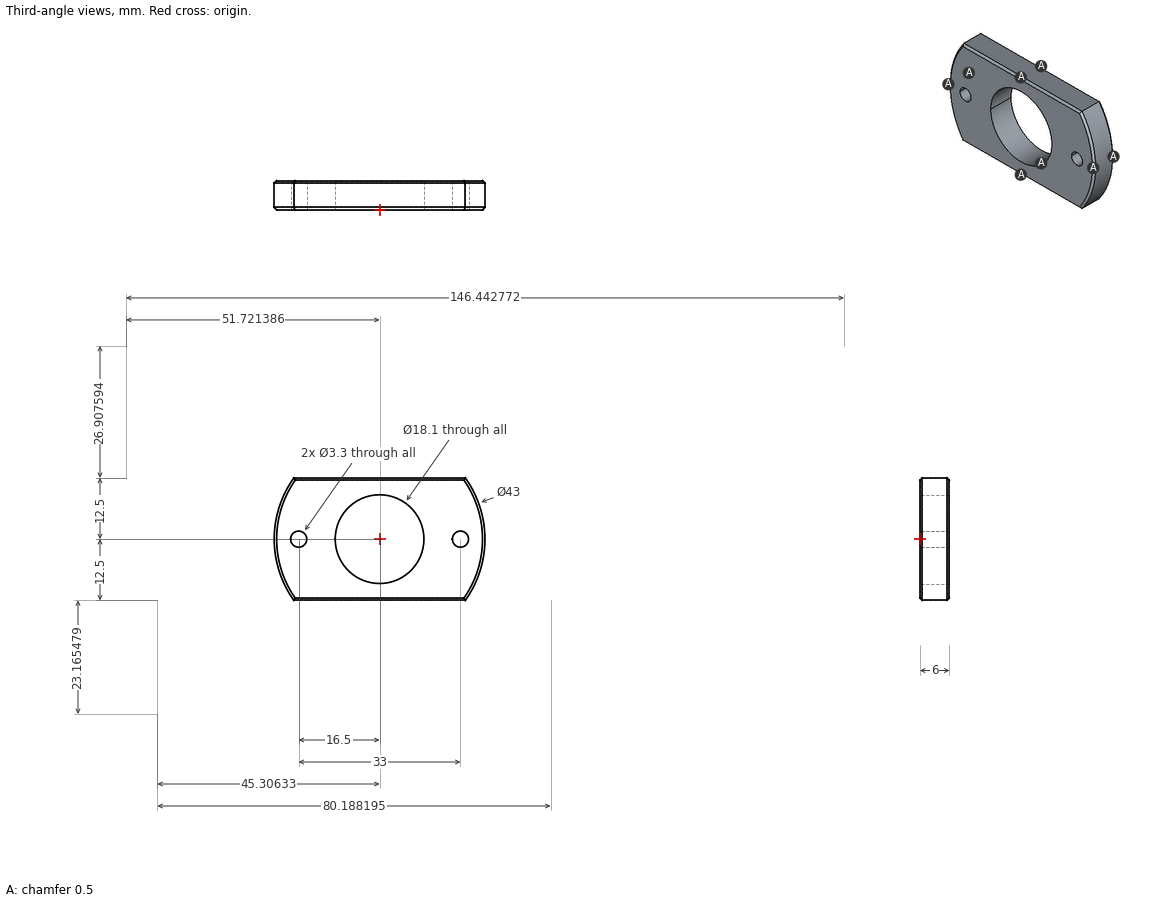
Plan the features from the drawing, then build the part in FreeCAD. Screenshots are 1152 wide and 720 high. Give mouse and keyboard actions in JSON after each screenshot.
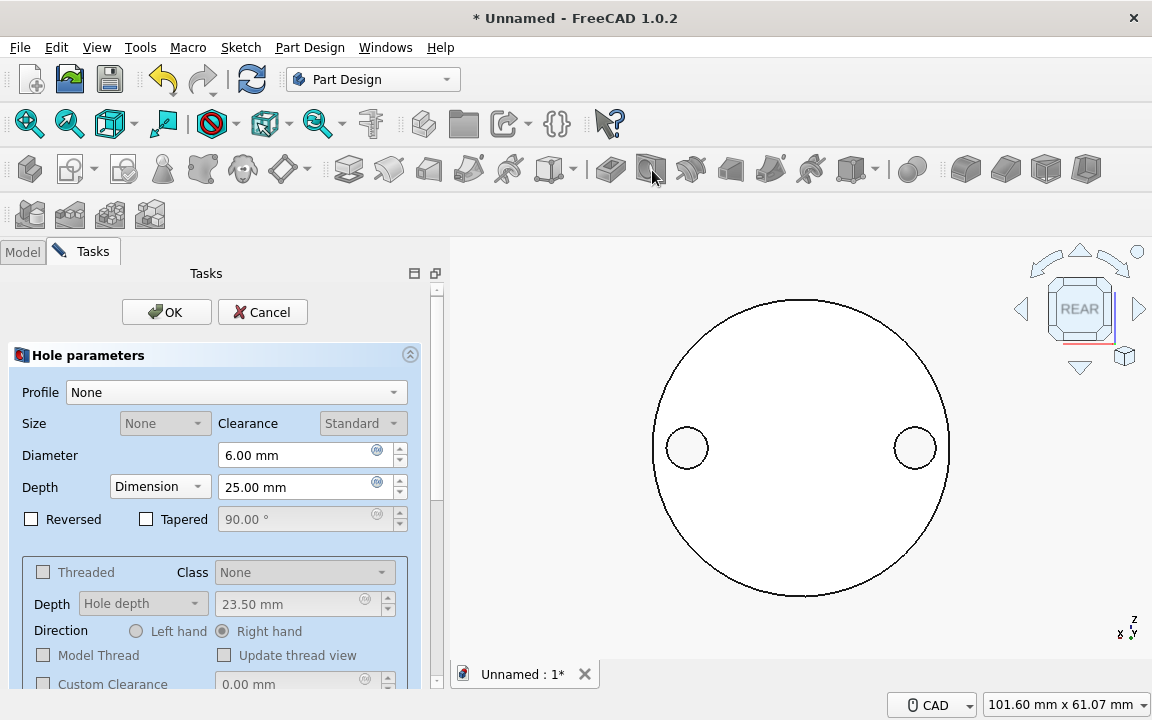
{"action": "triple_click", "coordinate": [305, 455]}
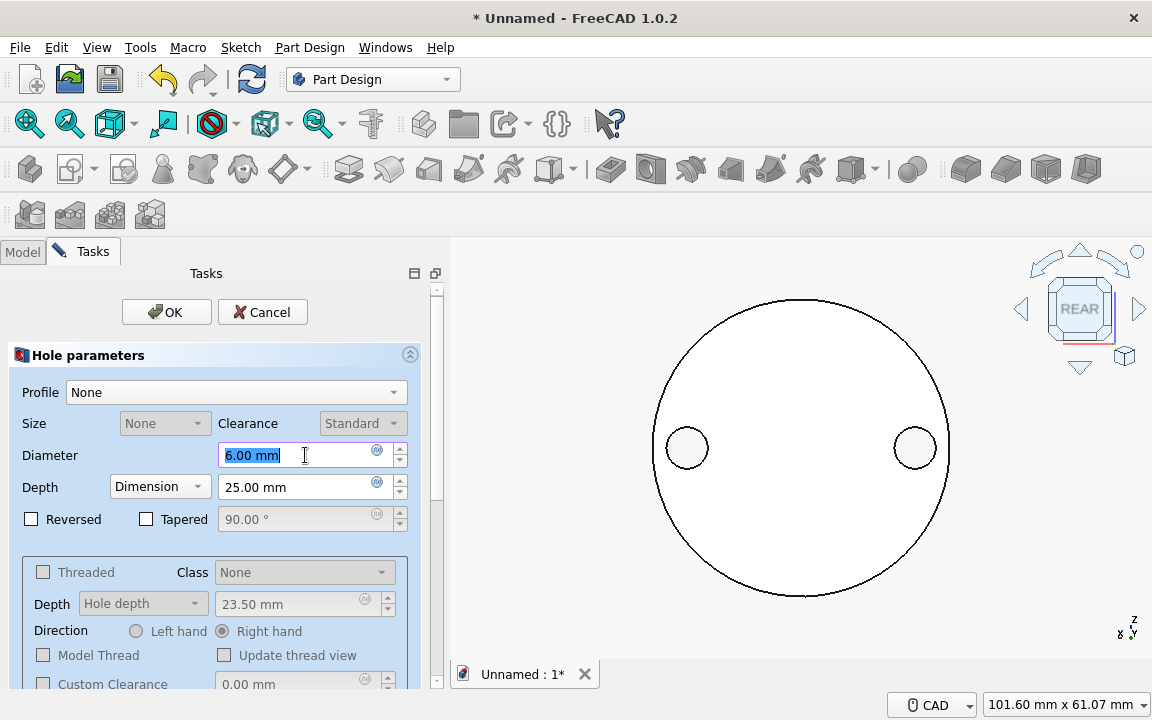
{"action": "type", "text": "3.3"}
{"action": "key", "text": "Tab"}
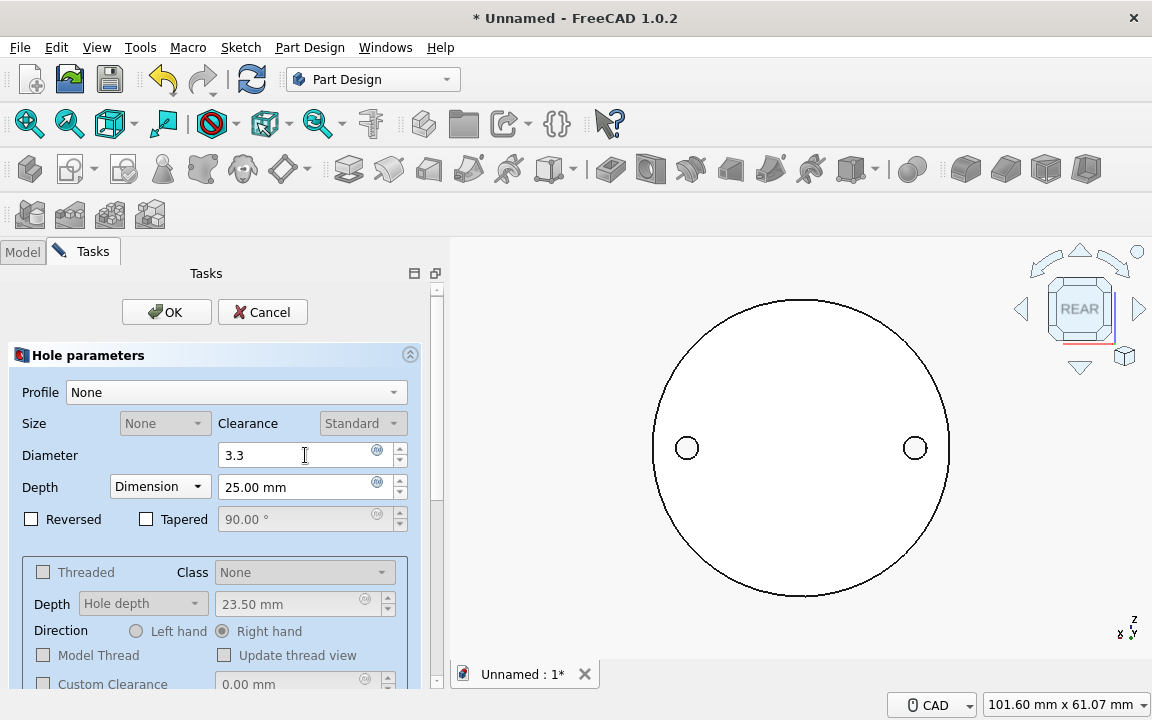
{"action": "left_click", "coordinate": [161, 486]}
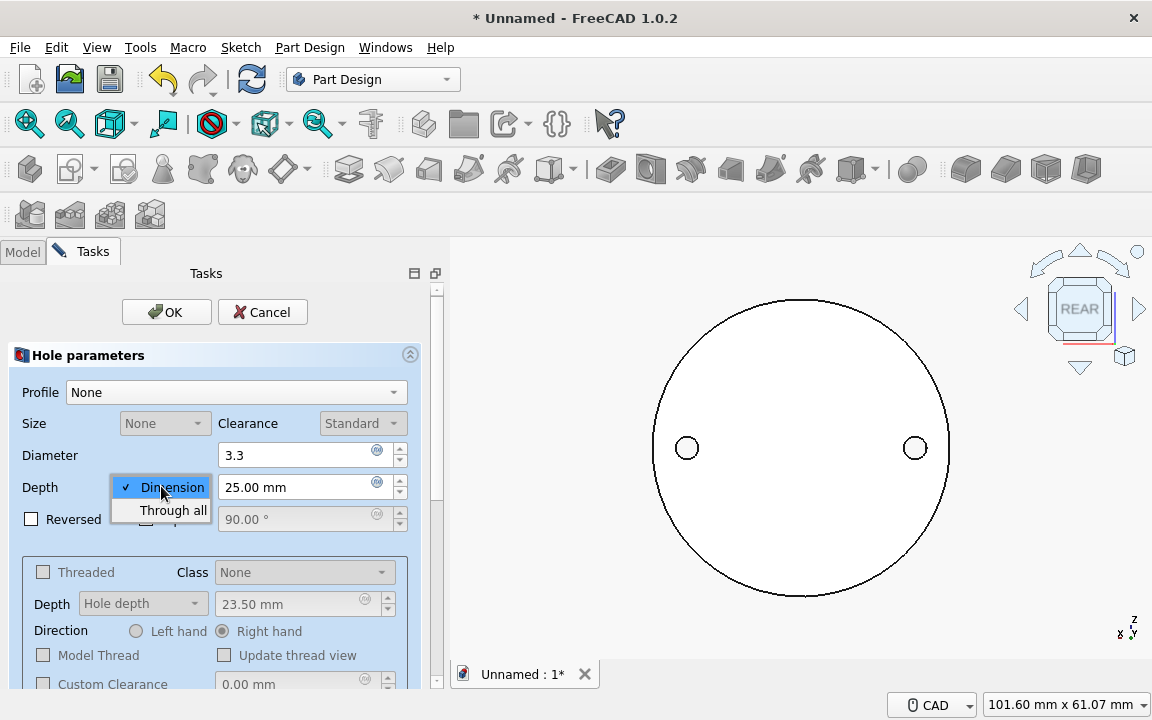
{"action": "left_click", "coordinate": [160, 510]}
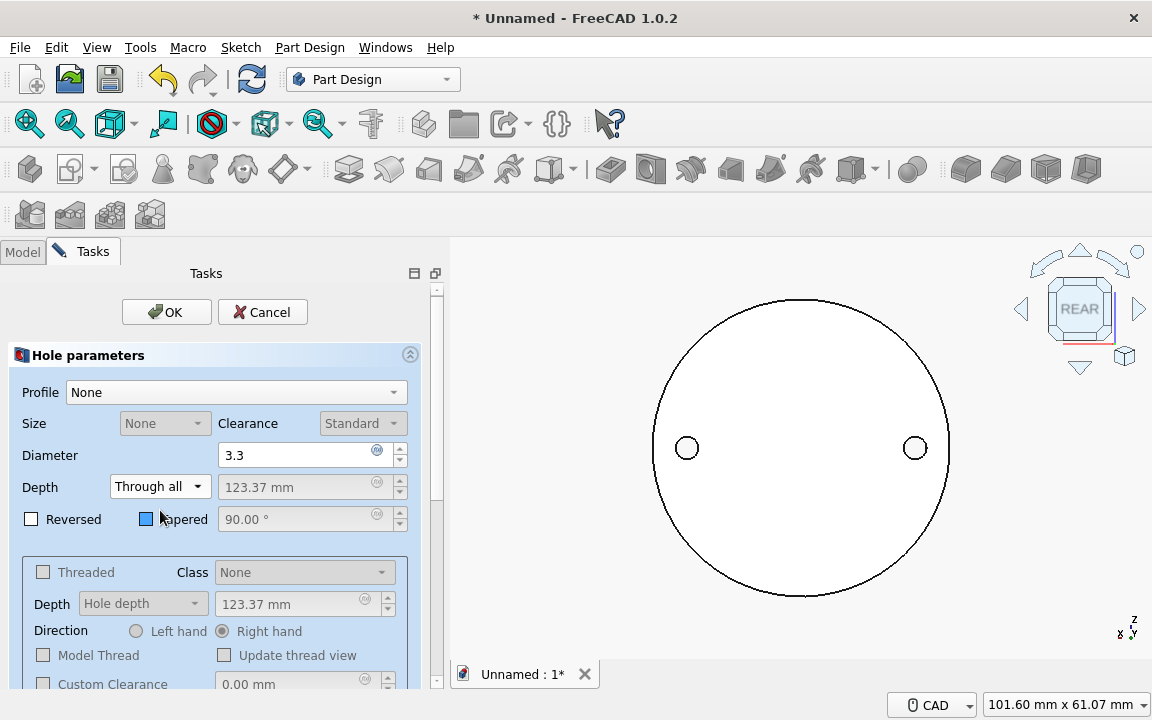
{"action": "left_click", "coordinate": [167, 312]}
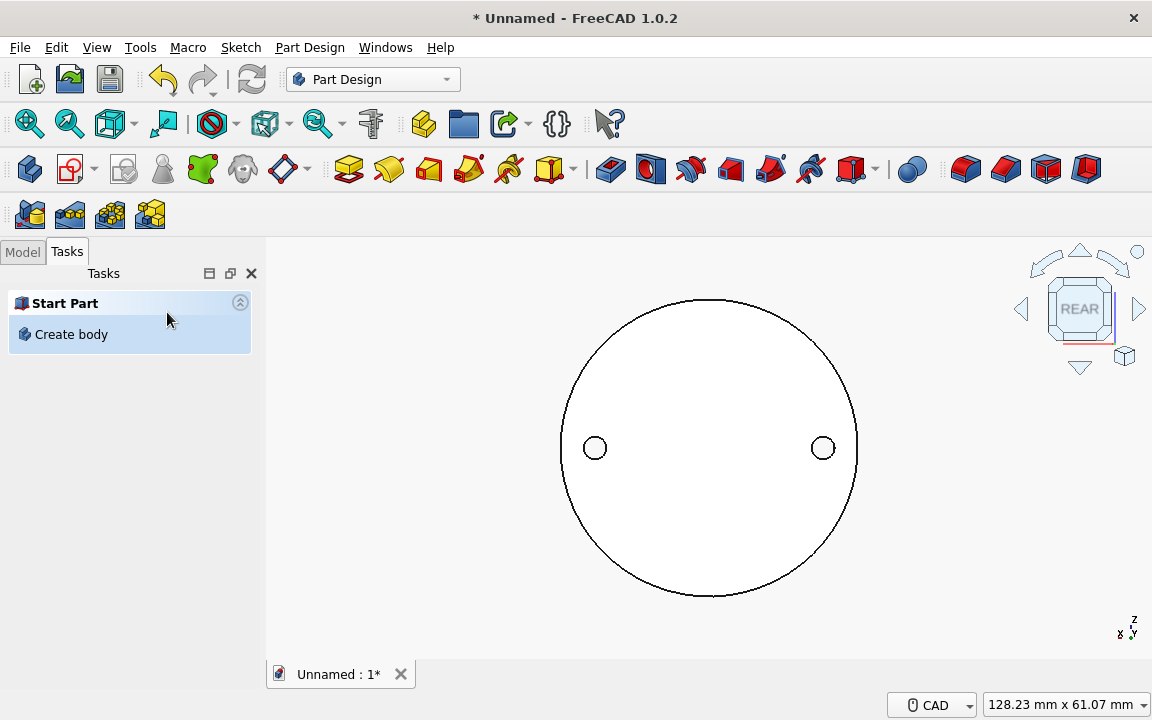
{"action": "left_click", "coordinate": [709, 405]}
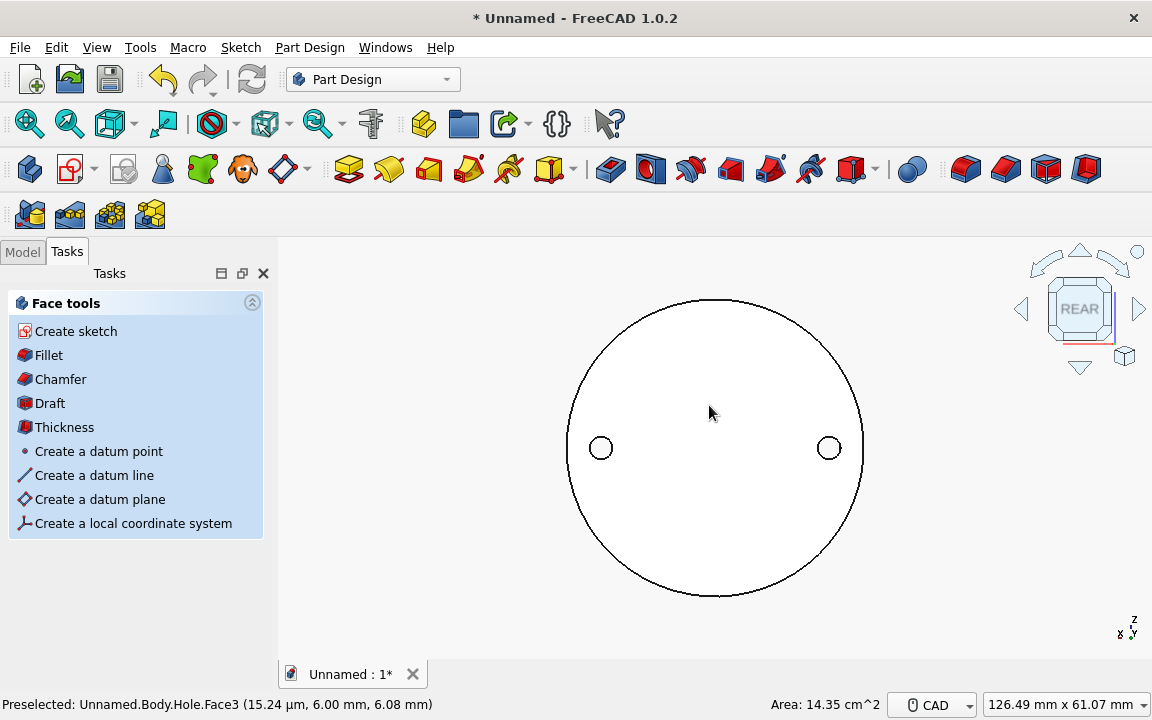
{"action": "left_click", "coordinate": [70, 170]}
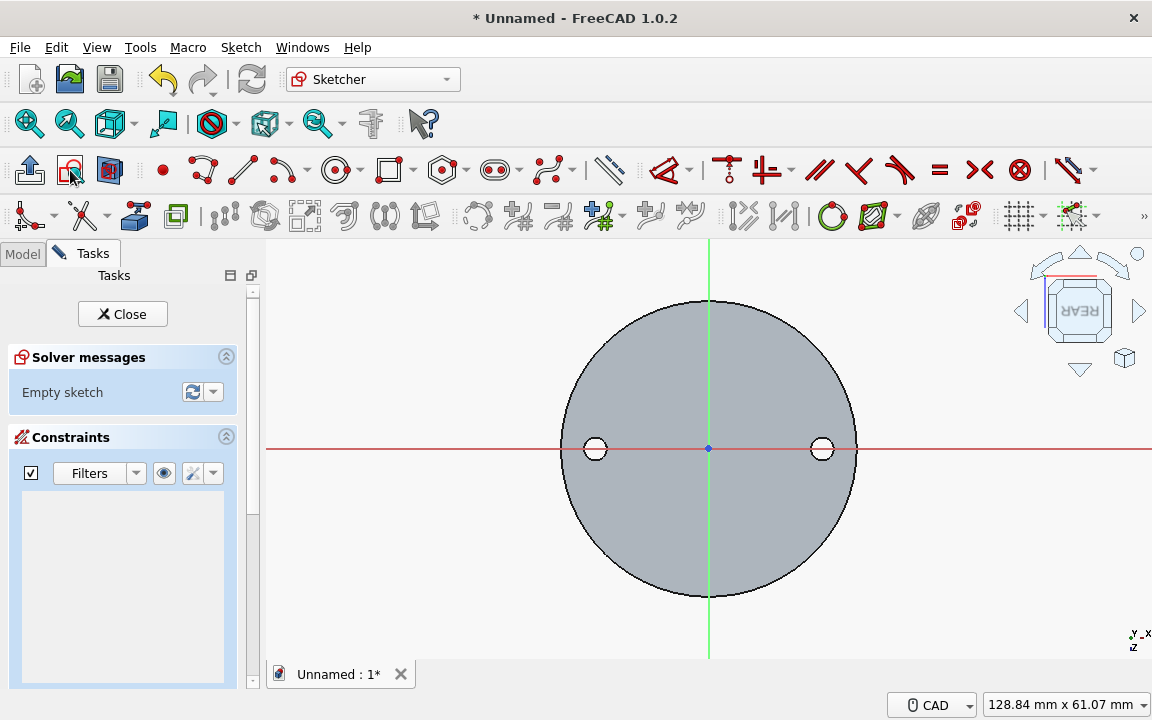
{"action": "scroll", "coordinate": [464, 439], "scroll_direction": "down", "scroll_amount": 4}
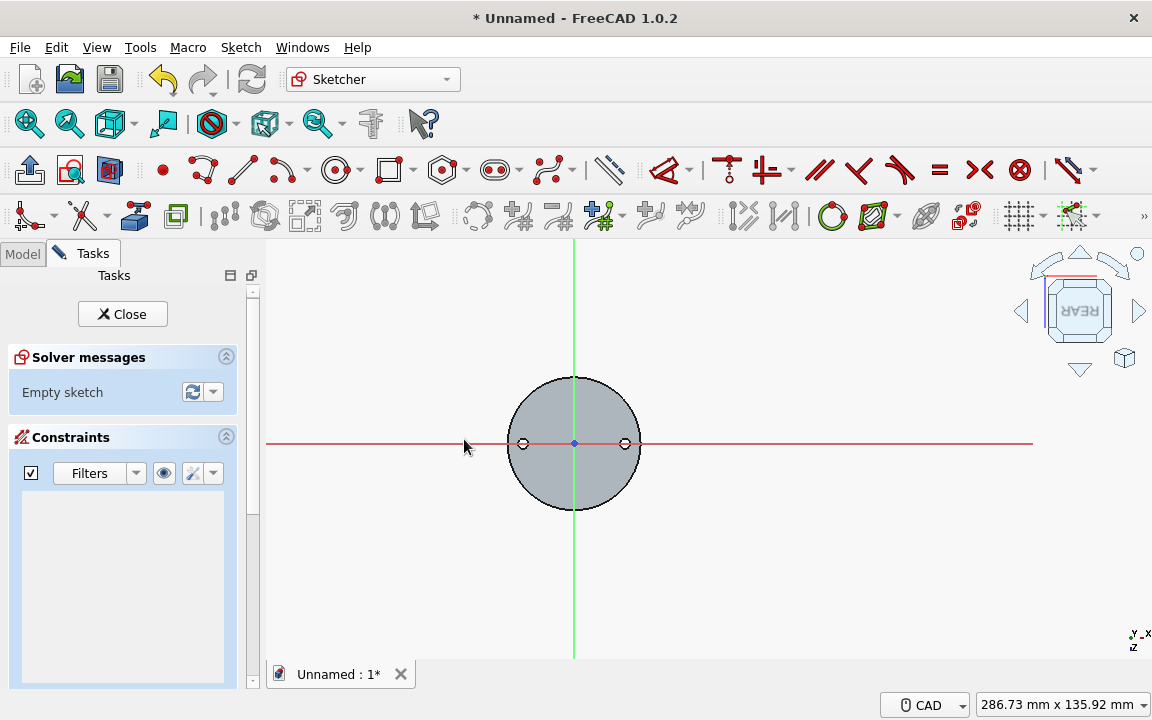
{"action": "left_click", "coordinate": [390, 170]}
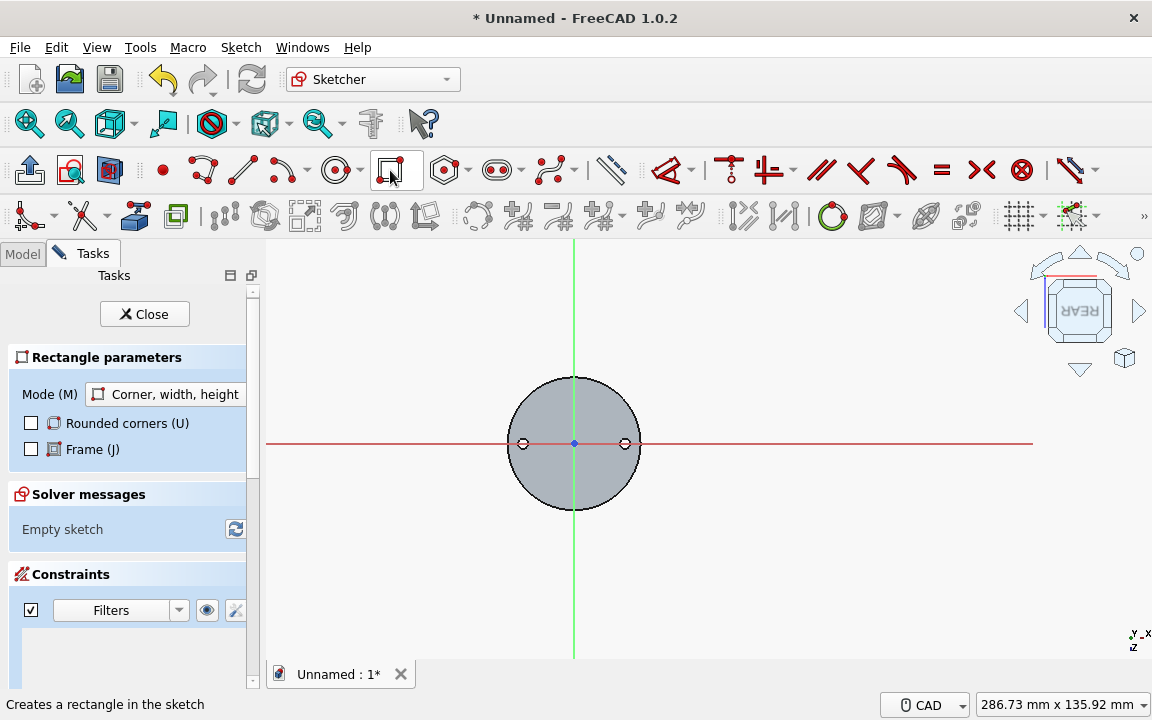
{"action": "left_click", "coordinate": [434, 334]}
{"action": "left_click", "coordinate": [682, 405]}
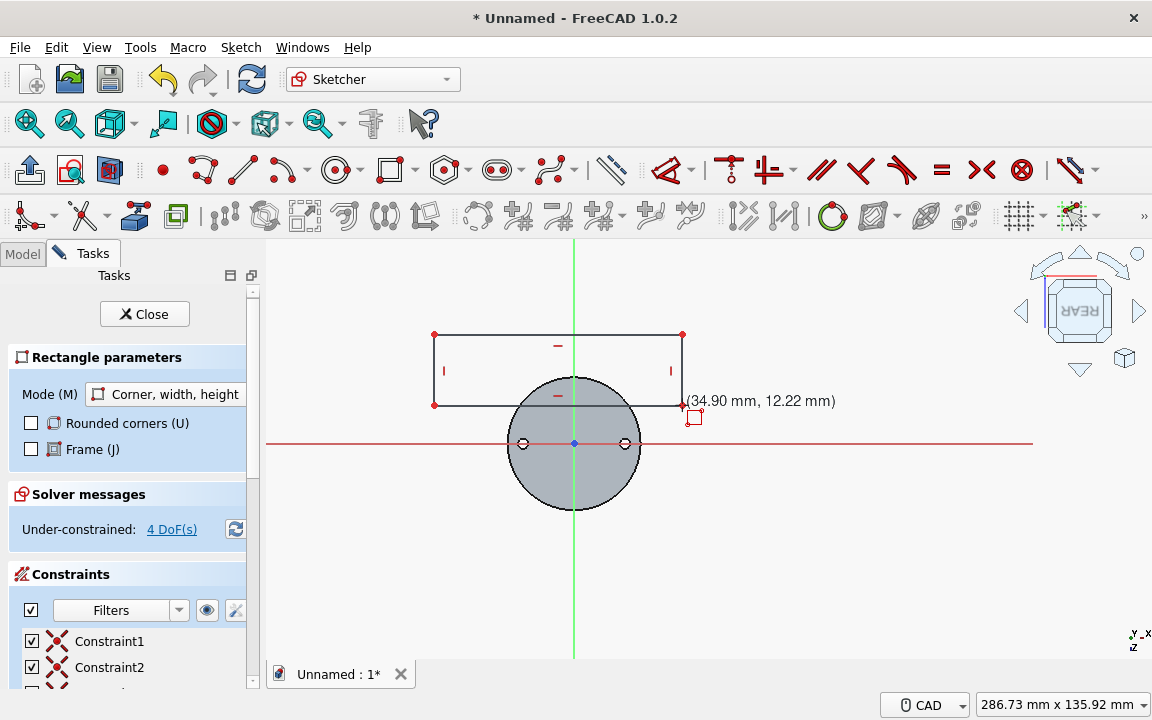
{"action": "left_click", "coordinate": [414, 482]}
{"action": "left_click", "coordinate": [867, 566]}
{"action": "key", "text": "Escape"}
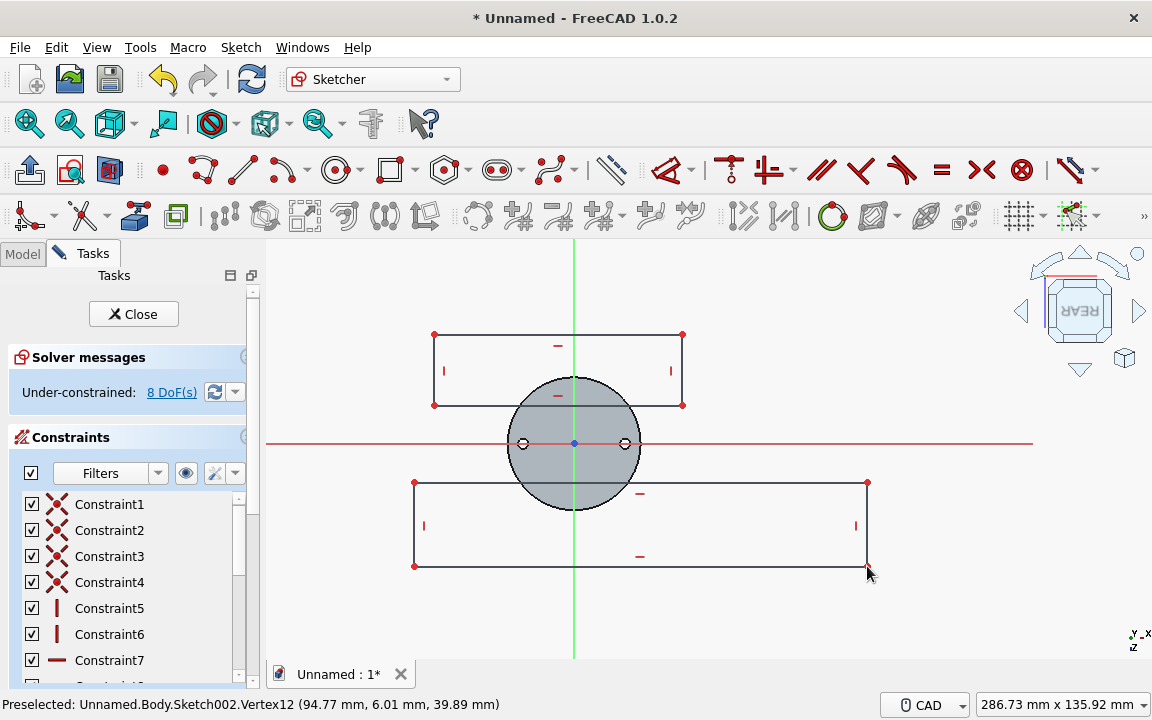
{"action": "left_click", "coordinate": [666, 170]}